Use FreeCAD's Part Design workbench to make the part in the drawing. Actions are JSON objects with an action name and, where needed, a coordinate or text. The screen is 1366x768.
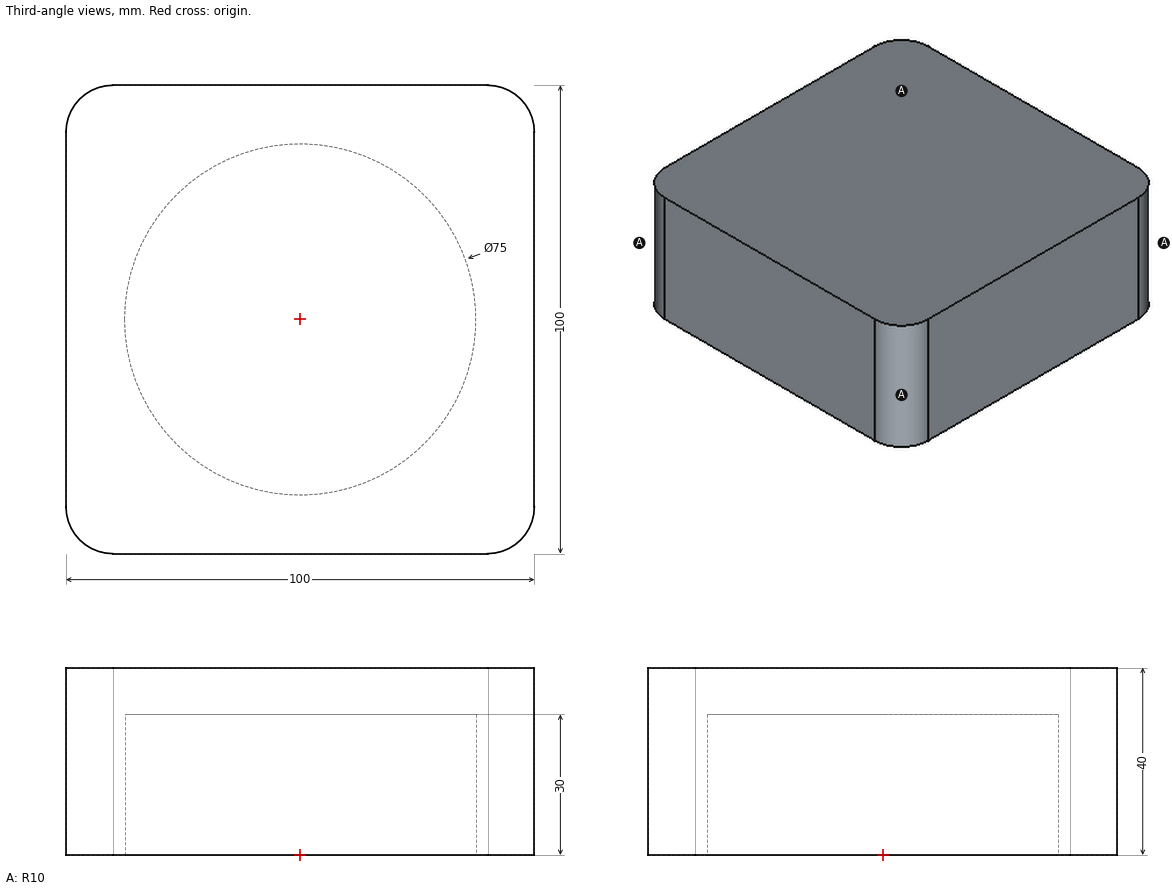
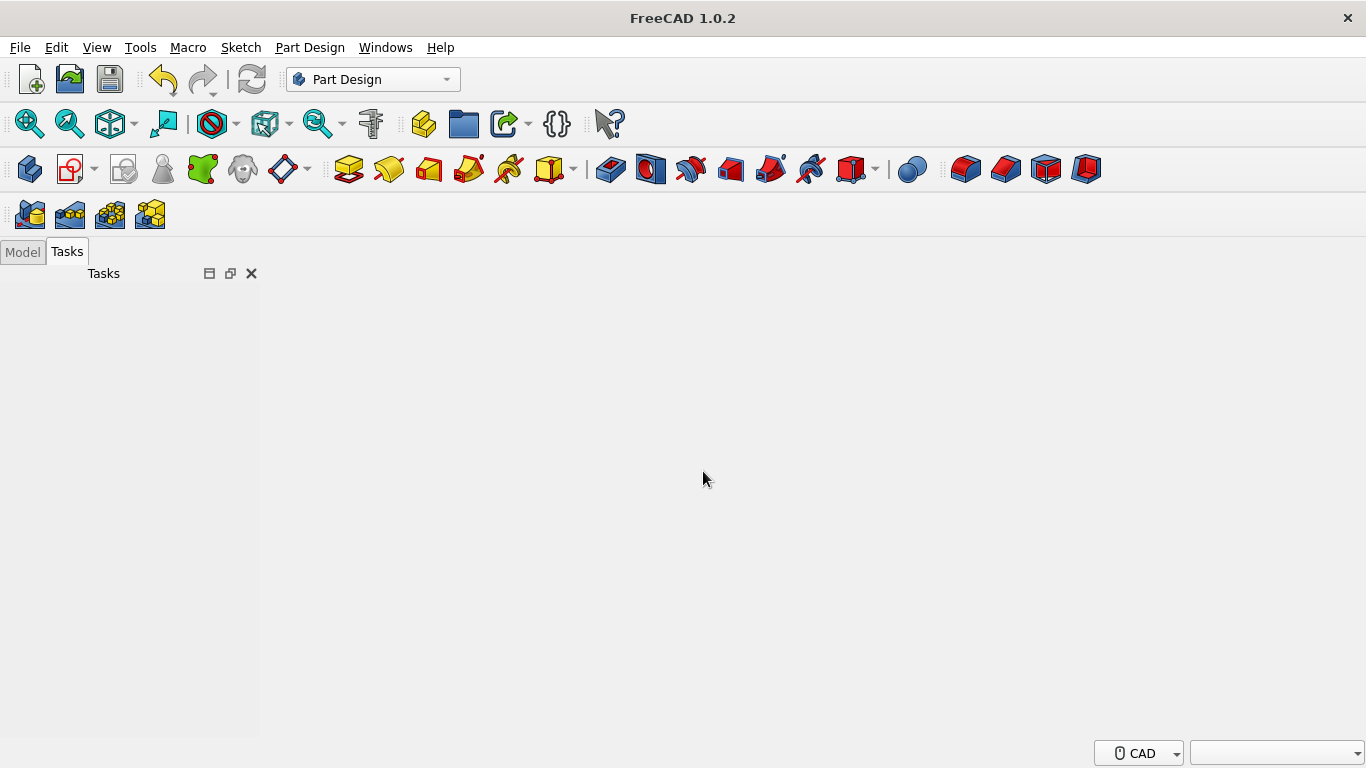
{"action": "key", "text": "ctrl+n"}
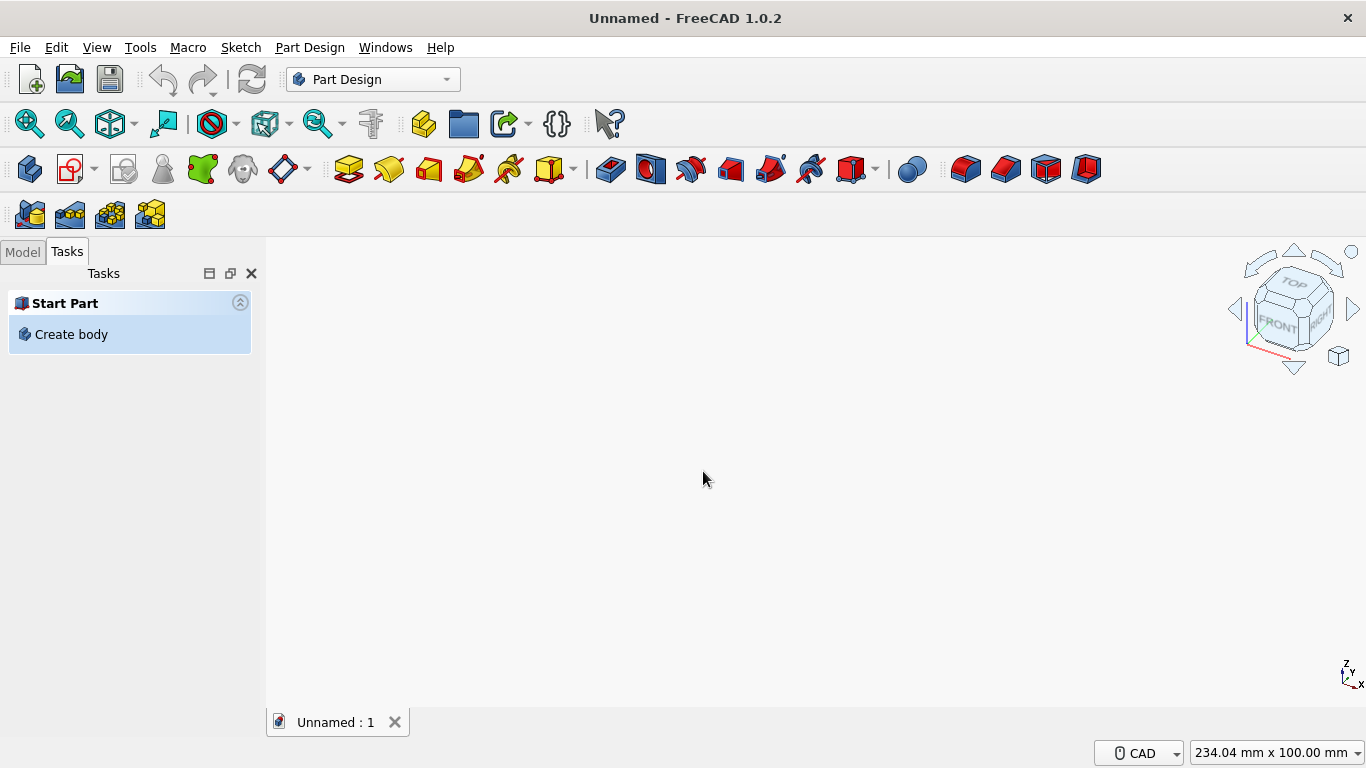
{"action": "left_click", "coordinate": [70, 170]}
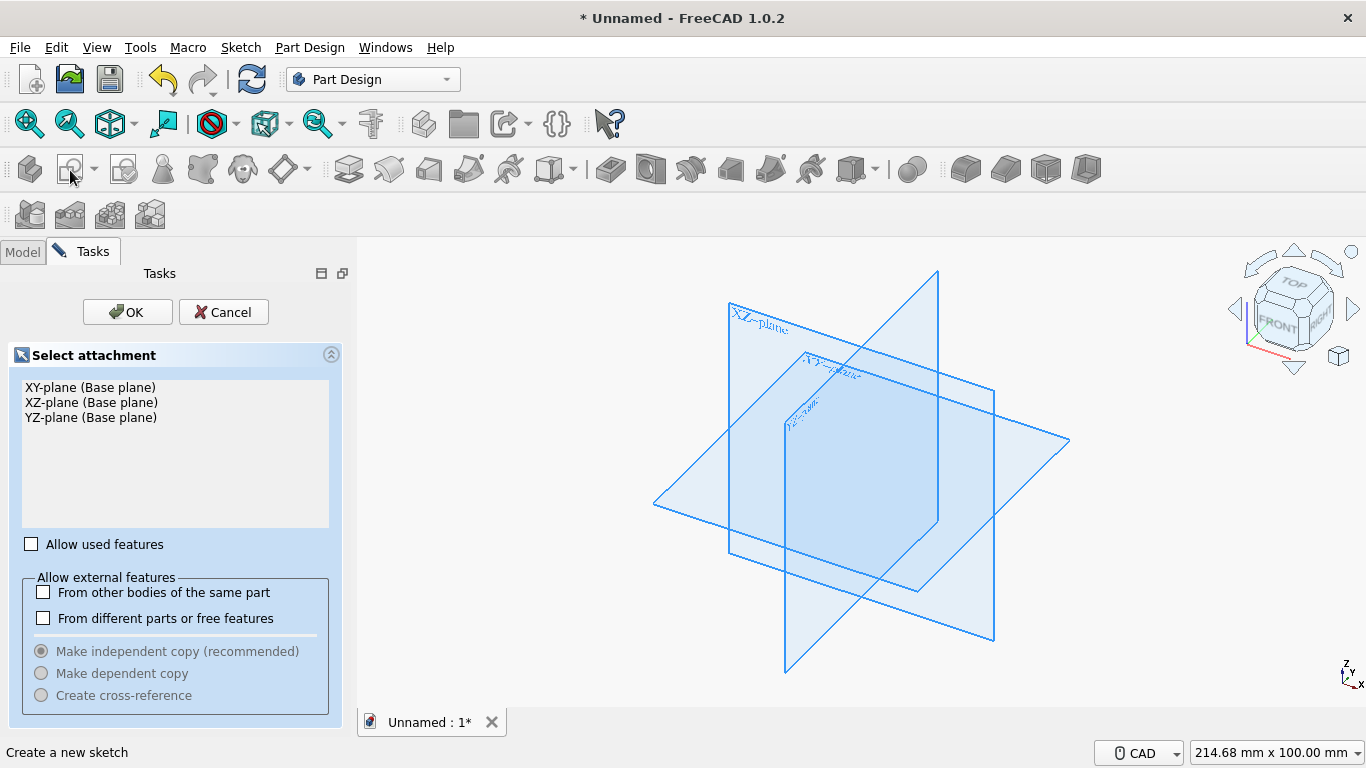
{"action": "left_click", "coordinate": [82, 388]}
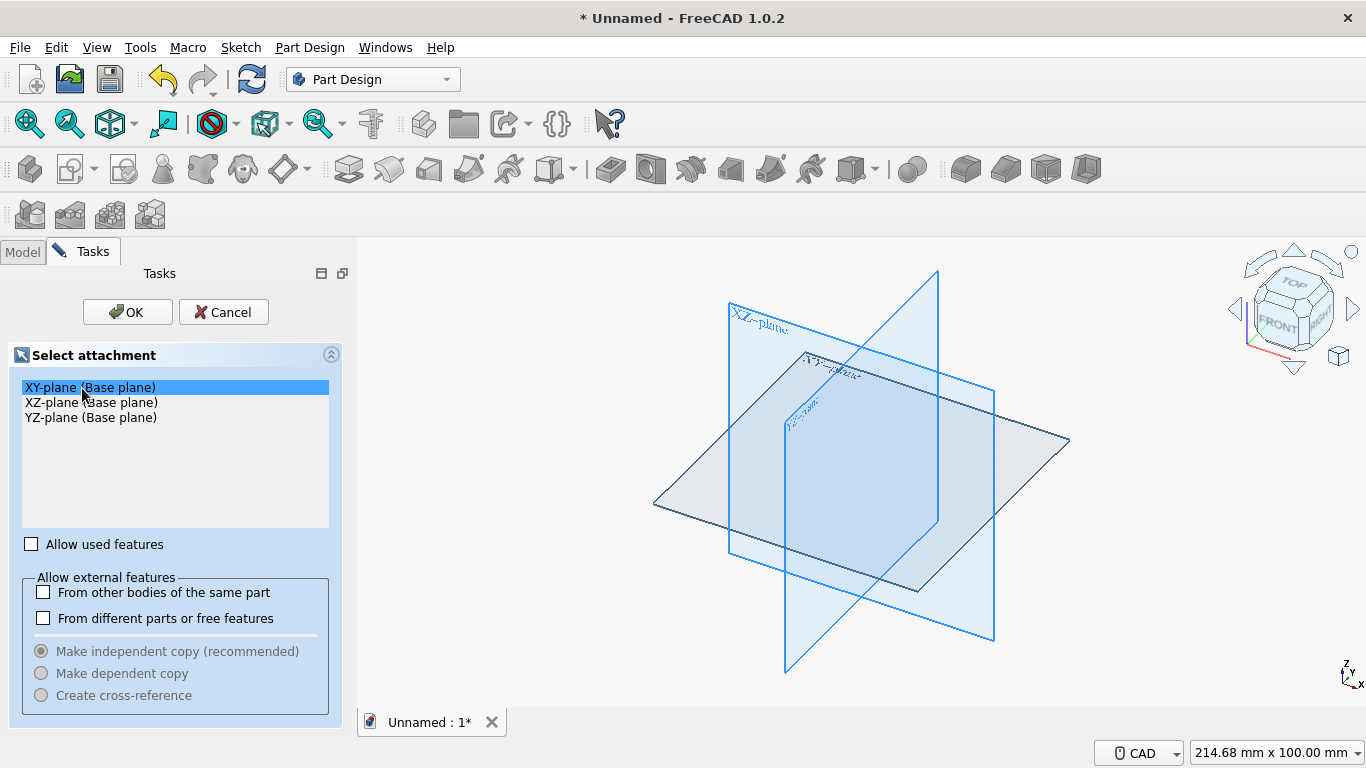
{"action": "left_click", "coordinate": [128, 312]}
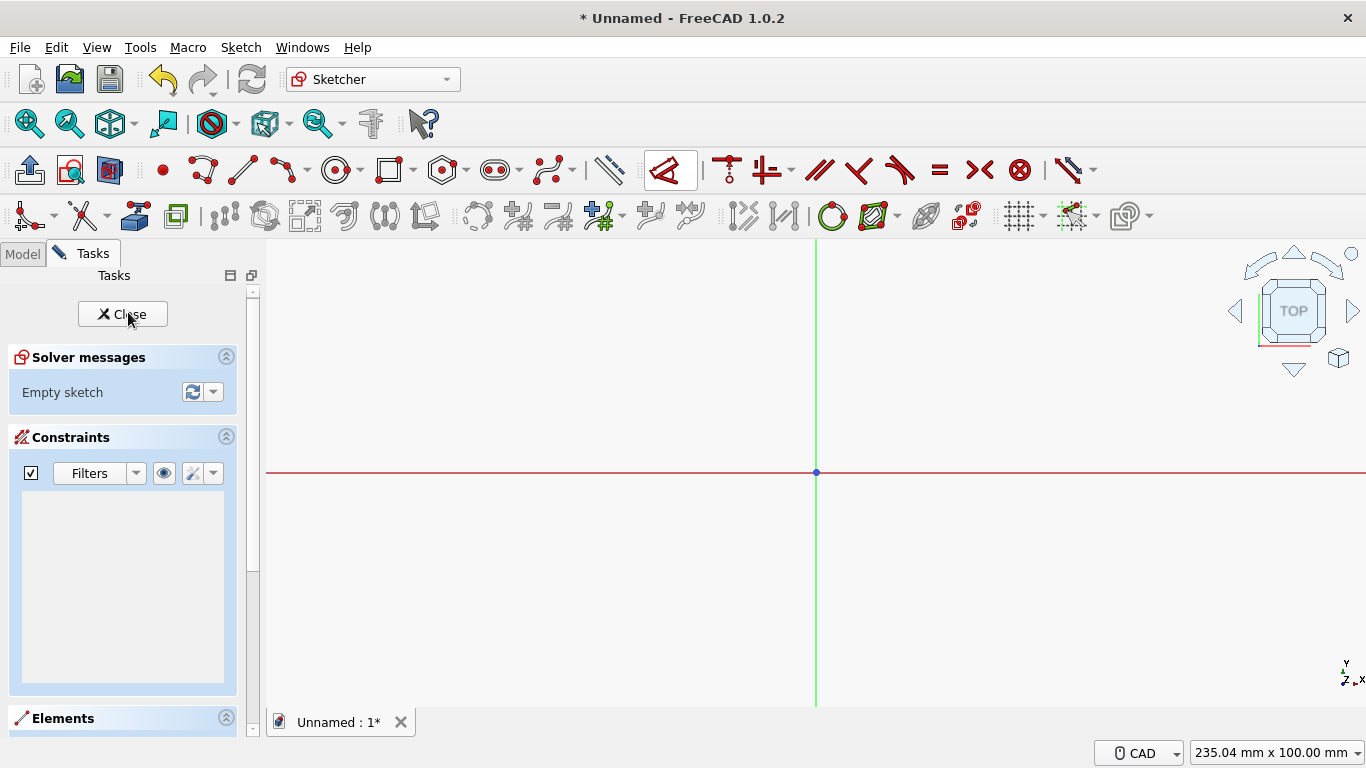
{"action": "scroll", "coordinate": [608, 473], "scroll_direction": "down", "scroll_amount": 2}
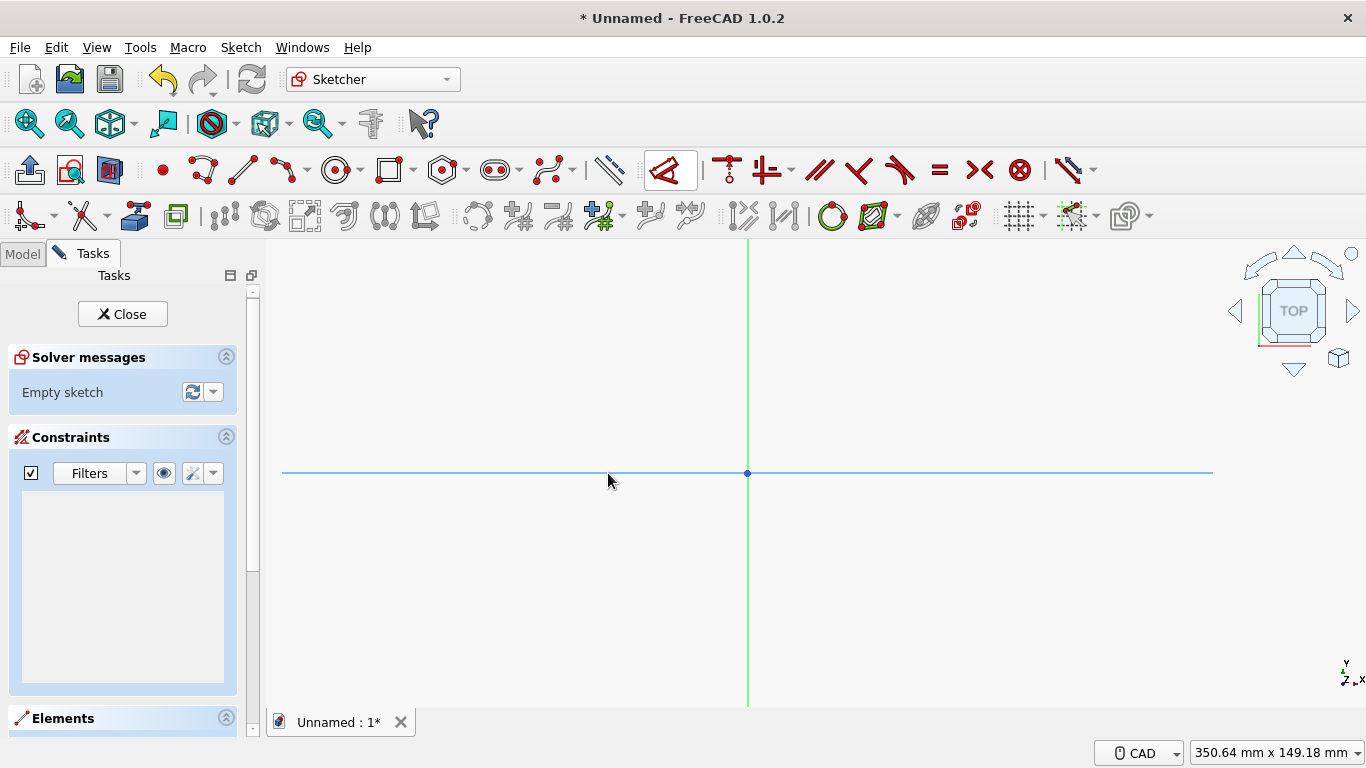
{"action": "left_click", "coordinate": [416, 170]}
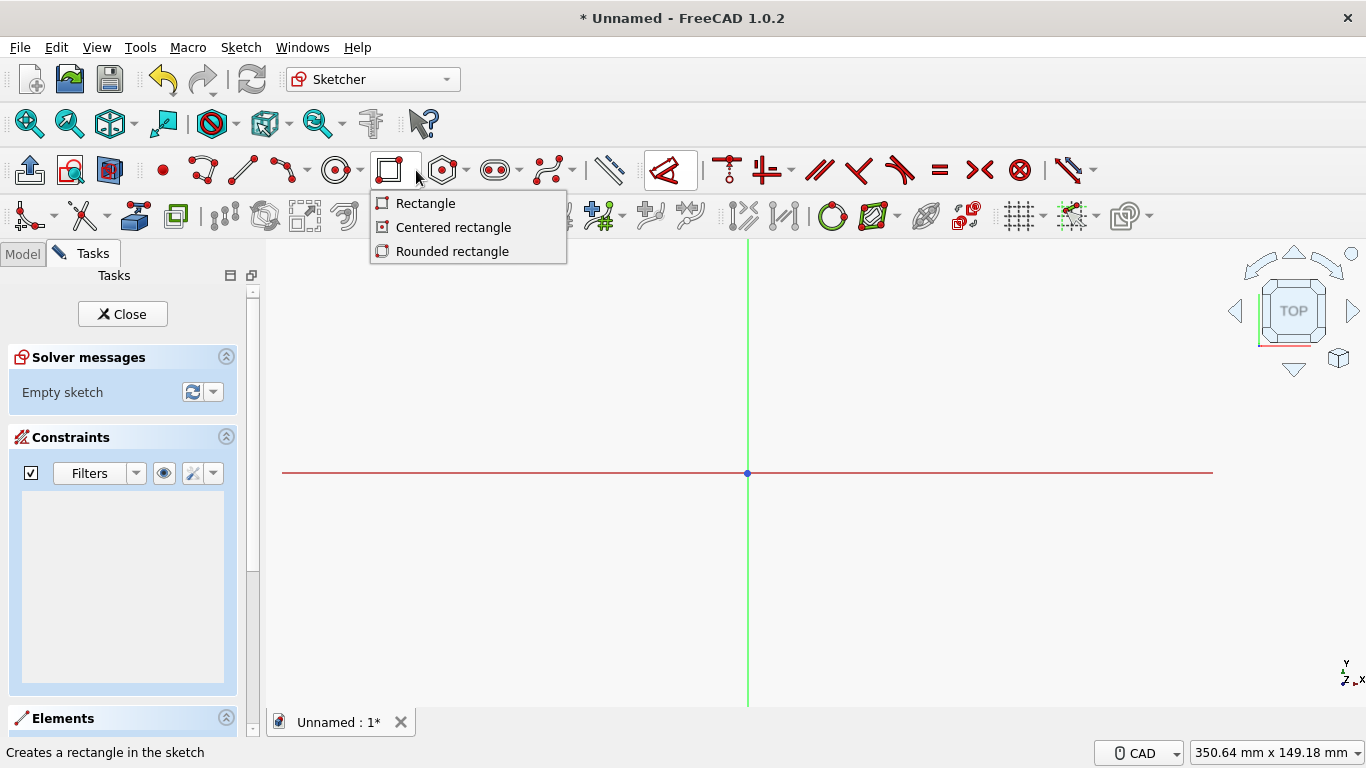
{"action": "left_click", "coordinate": [468, 227]}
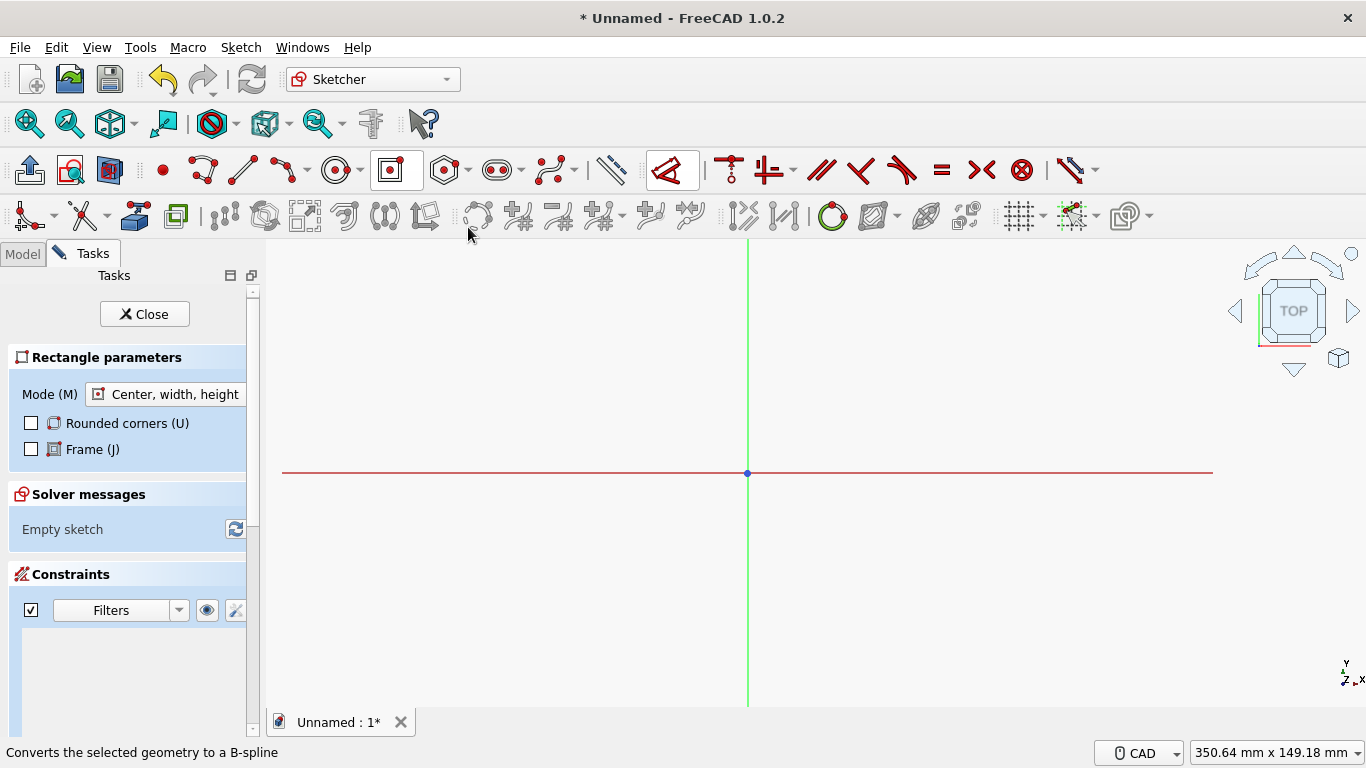
{"action": "left_click", "coordinate": [748, 473]}
{"action": "left_click", "coordinate": [904, 316]}
{"action": "key", "text": "Escape"}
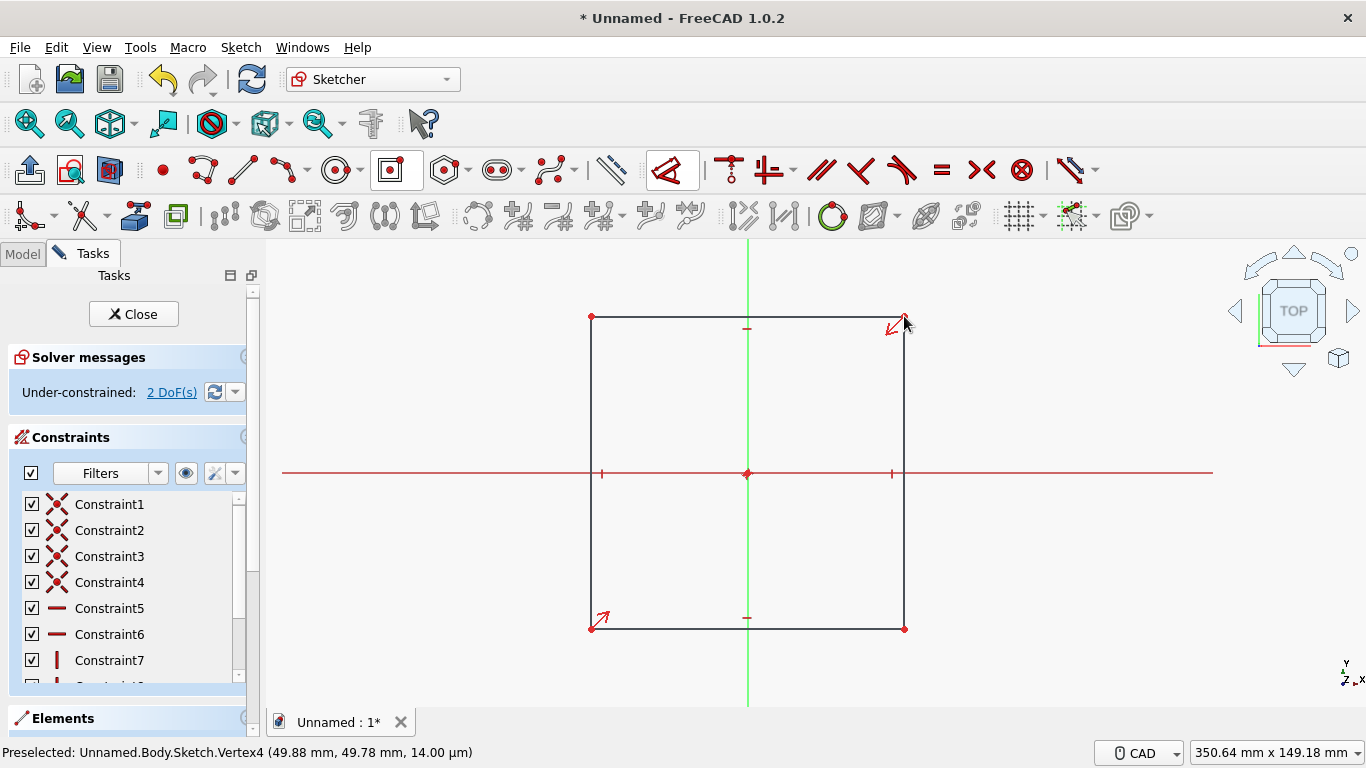
{"action": "key", "text": "d"}